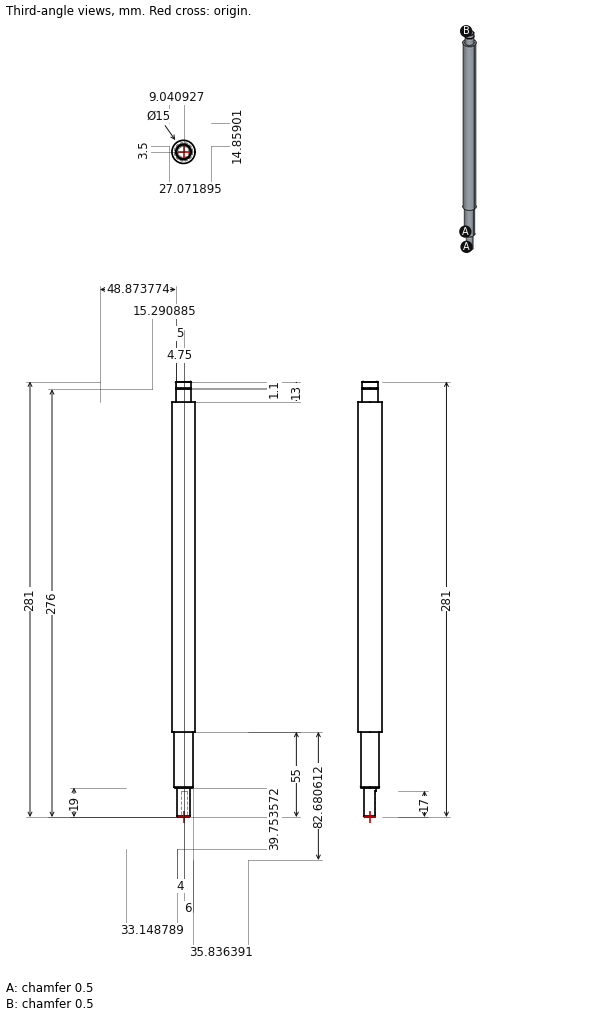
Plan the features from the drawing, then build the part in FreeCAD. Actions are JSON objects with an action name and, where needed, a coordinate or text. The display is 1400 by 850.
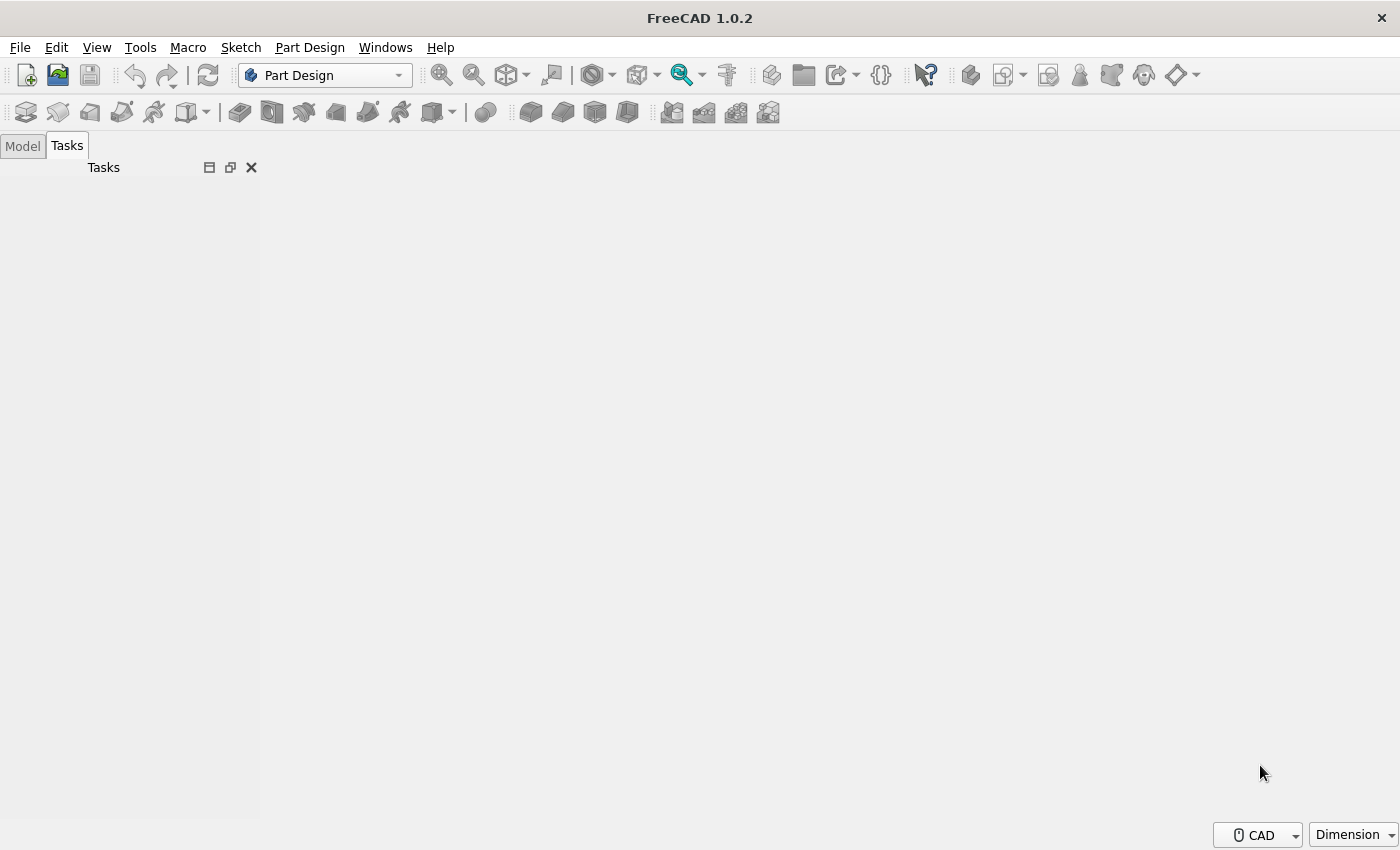
{"action": "left_click", "coordinate": [26, 76]}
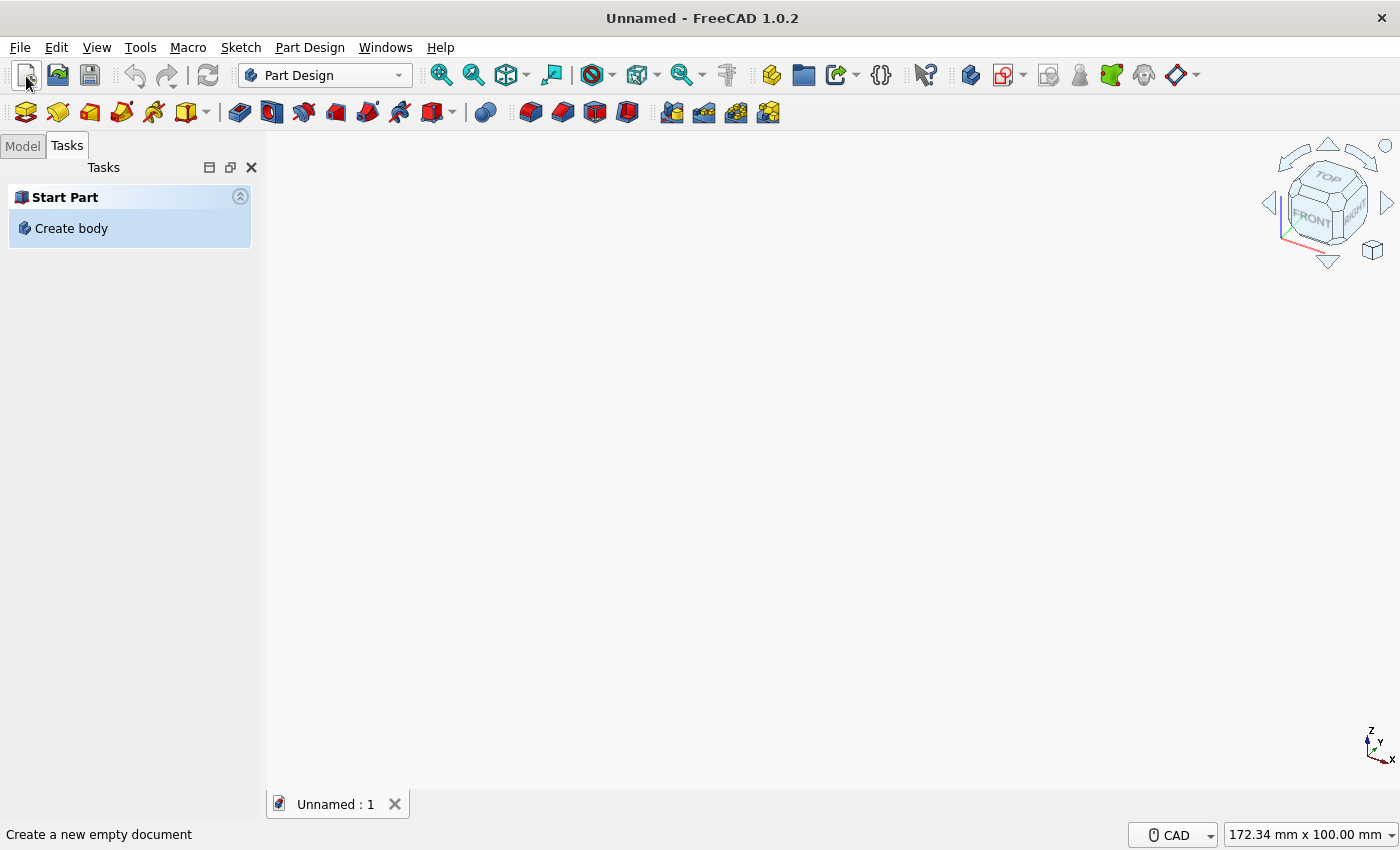
{"action": "left_click", "coordinate": [1004, 76]}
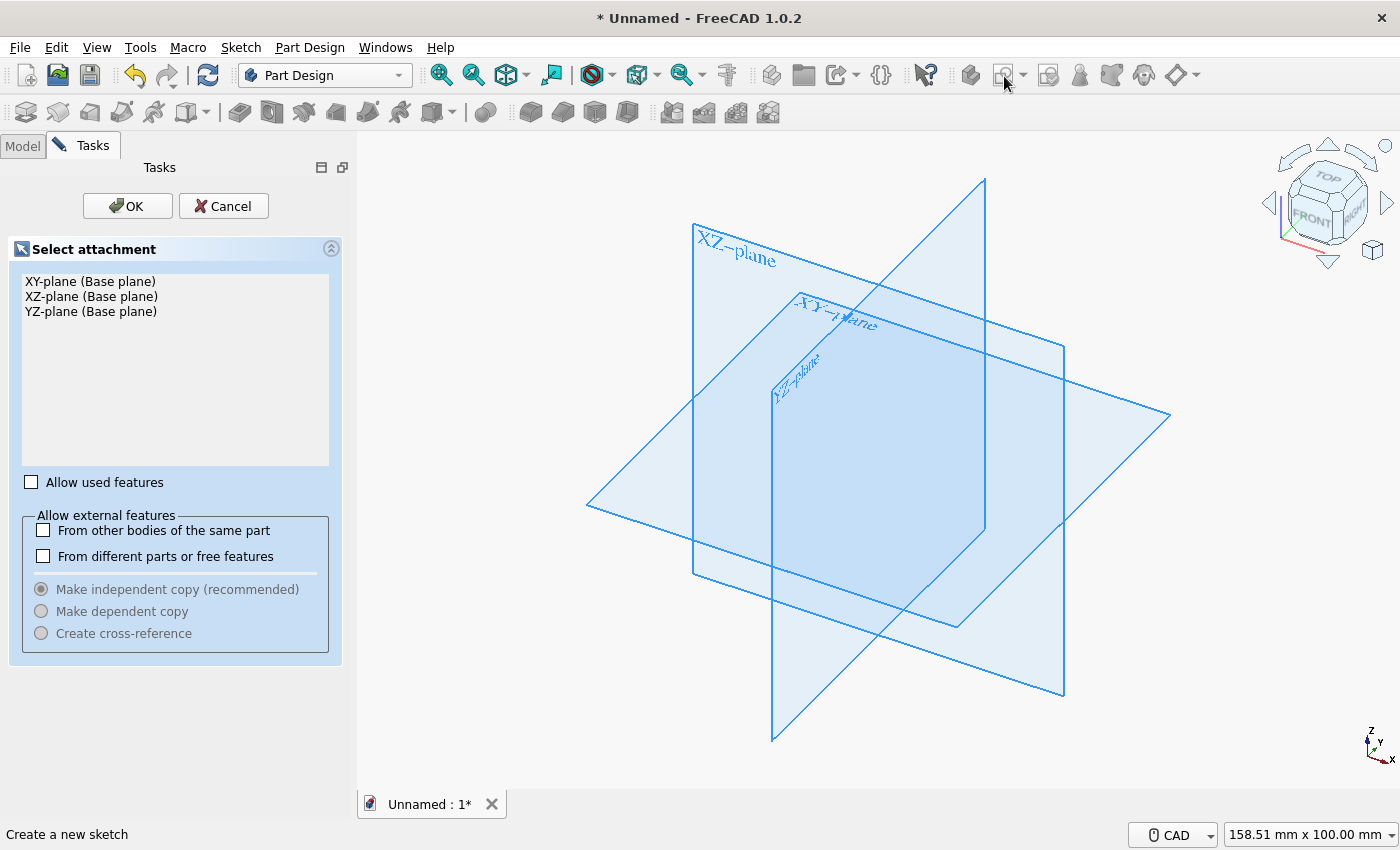
{"action": "left_click", "coordinate": [82, 282]}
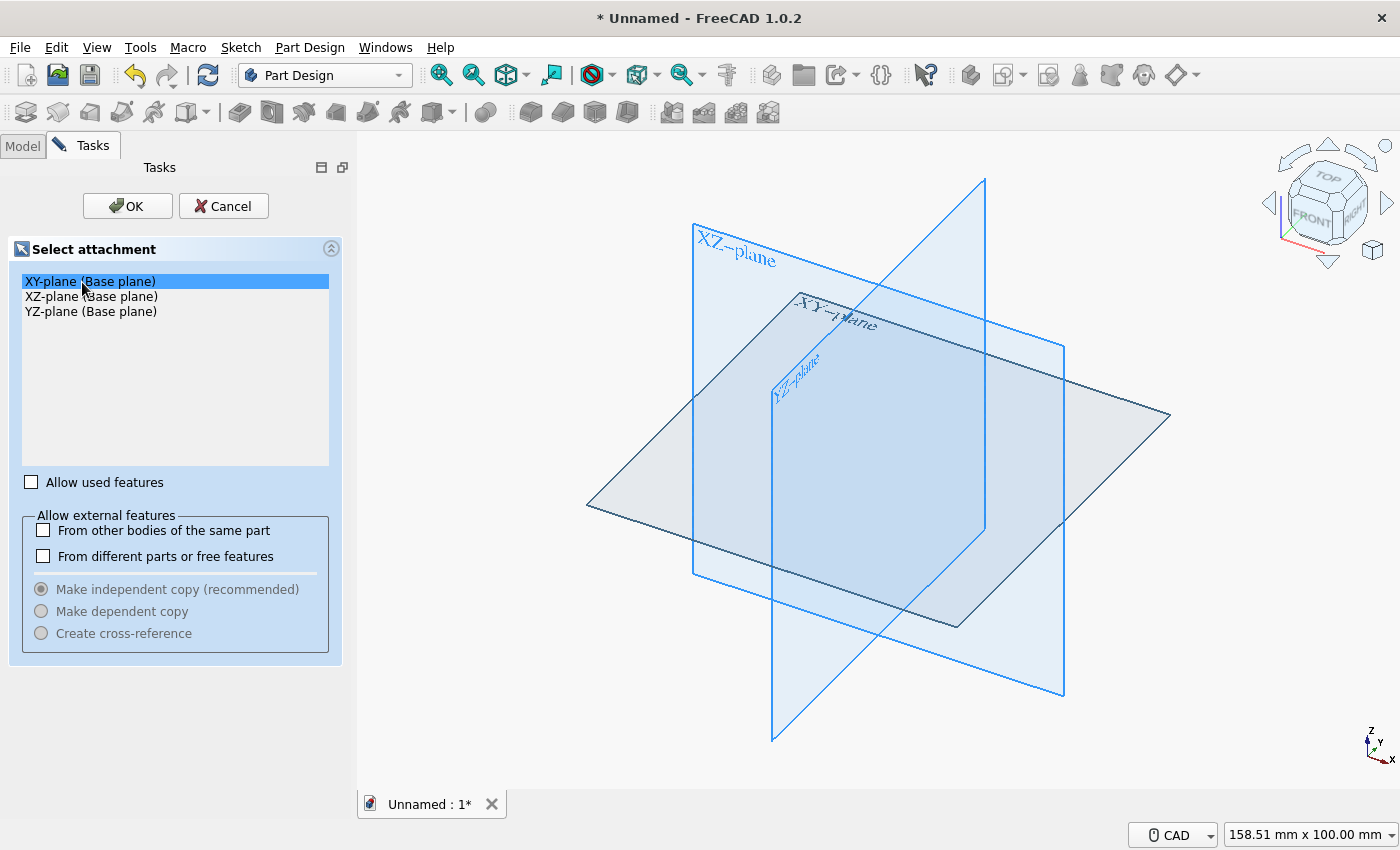
{"action": "left_click", "coordinate": [128, 206]}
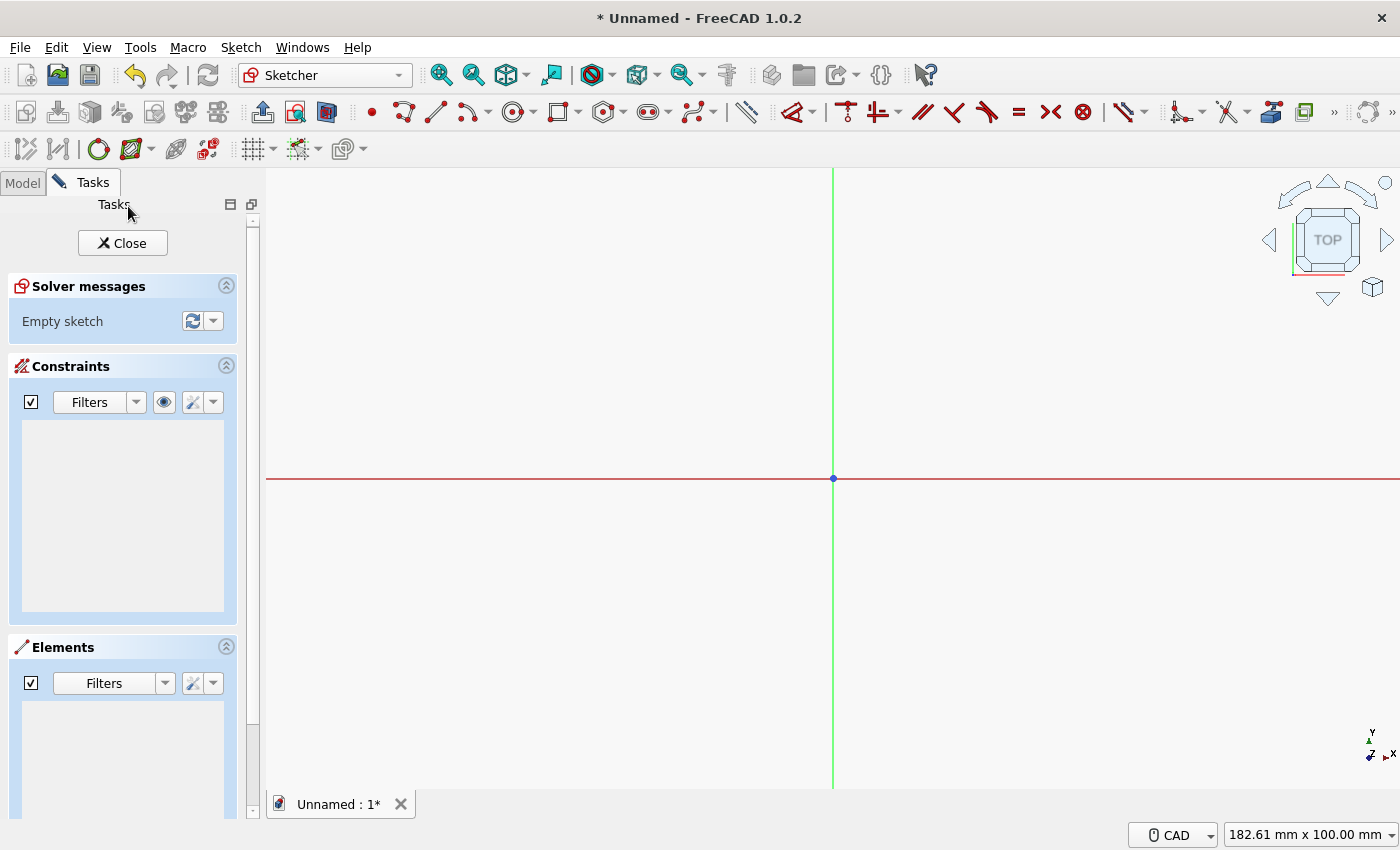
{"action": "scroll", "coordinate": [855, 479], "scroll_direction": "up", "scroll_amount": 7}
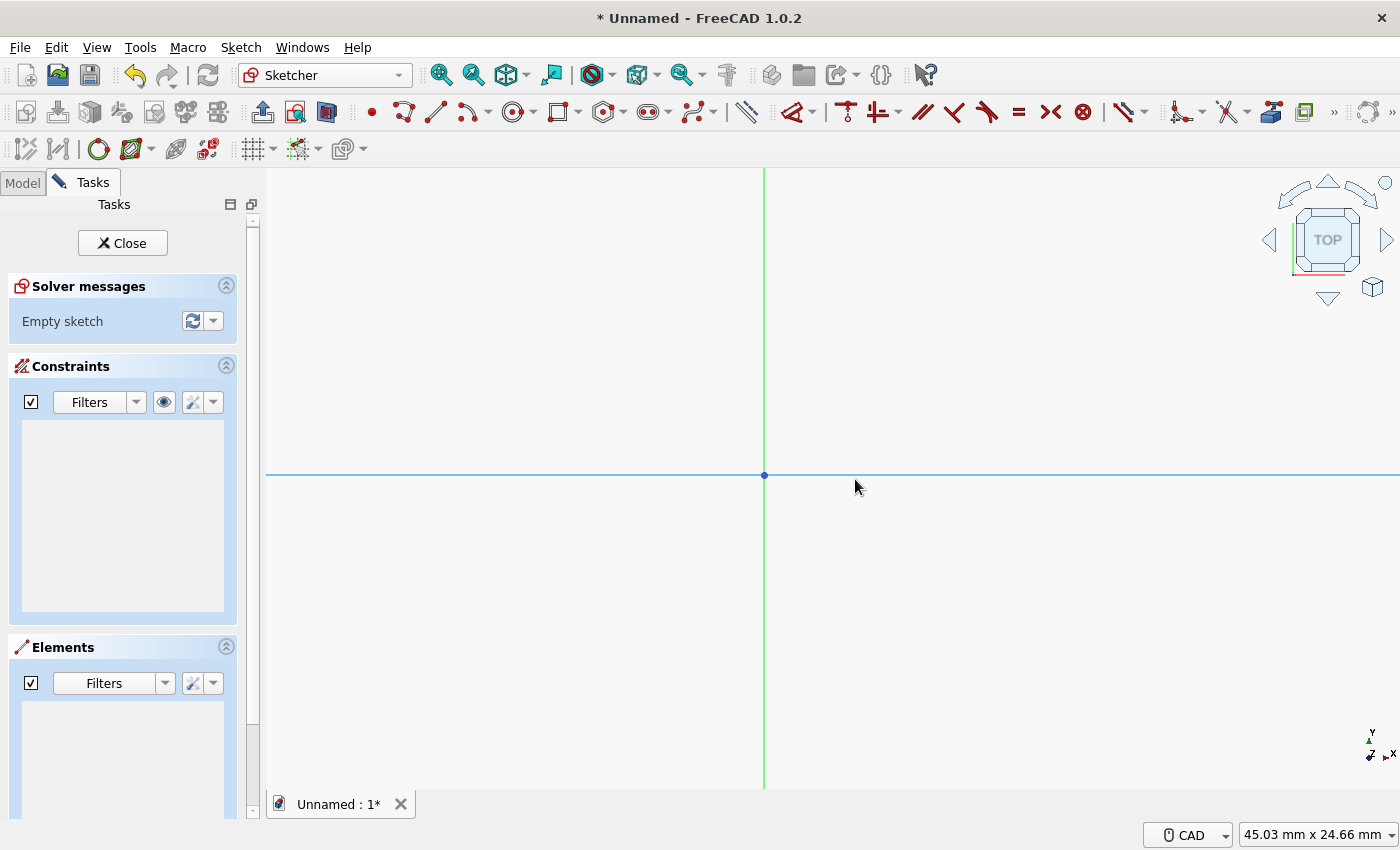
{"action": "left_click", "coordinate": [514, 112]}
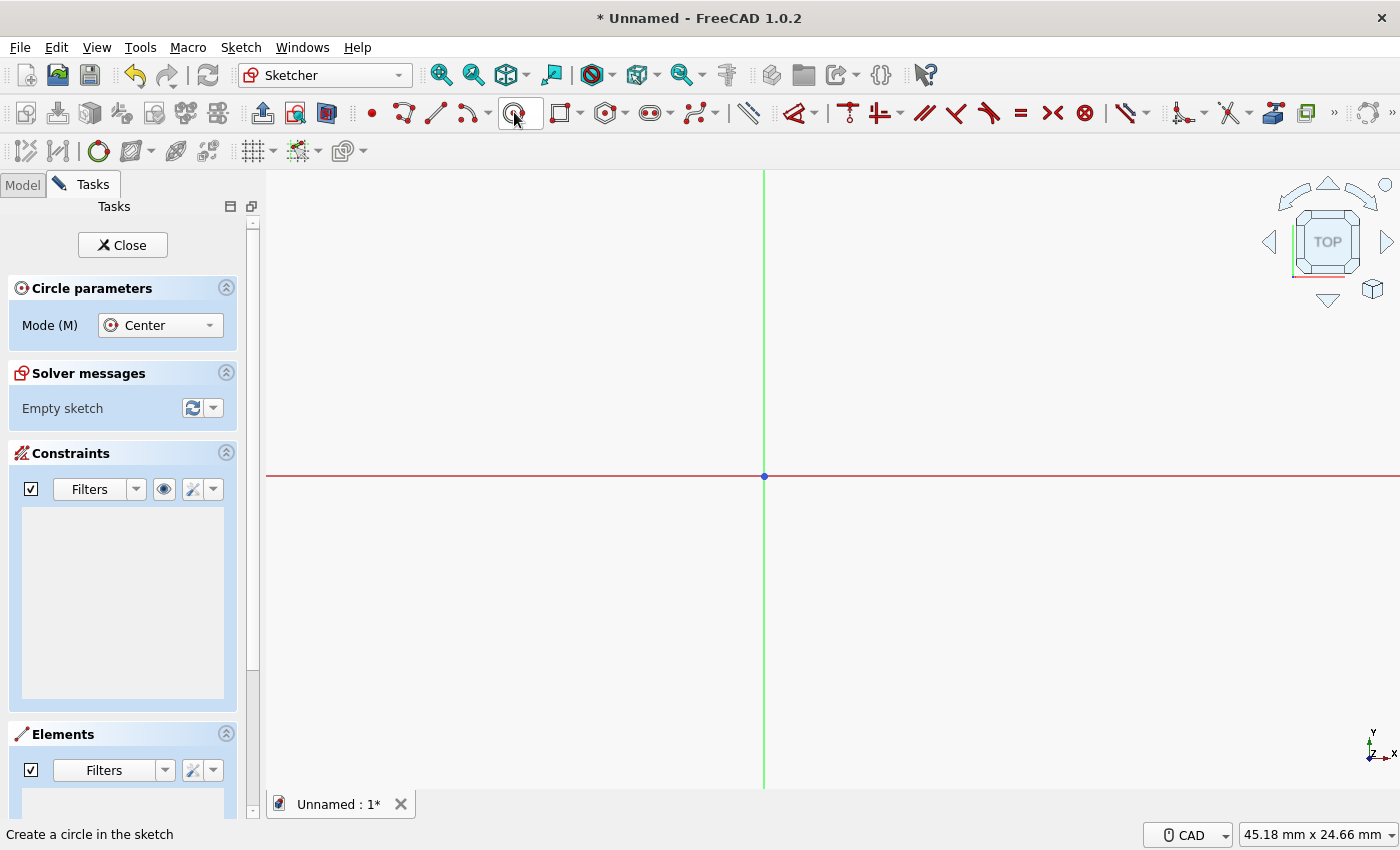
{"action": "left_click", "coordinate": [764, 476]}
{"action": "mouse_move", "coordinate": [898, 343]}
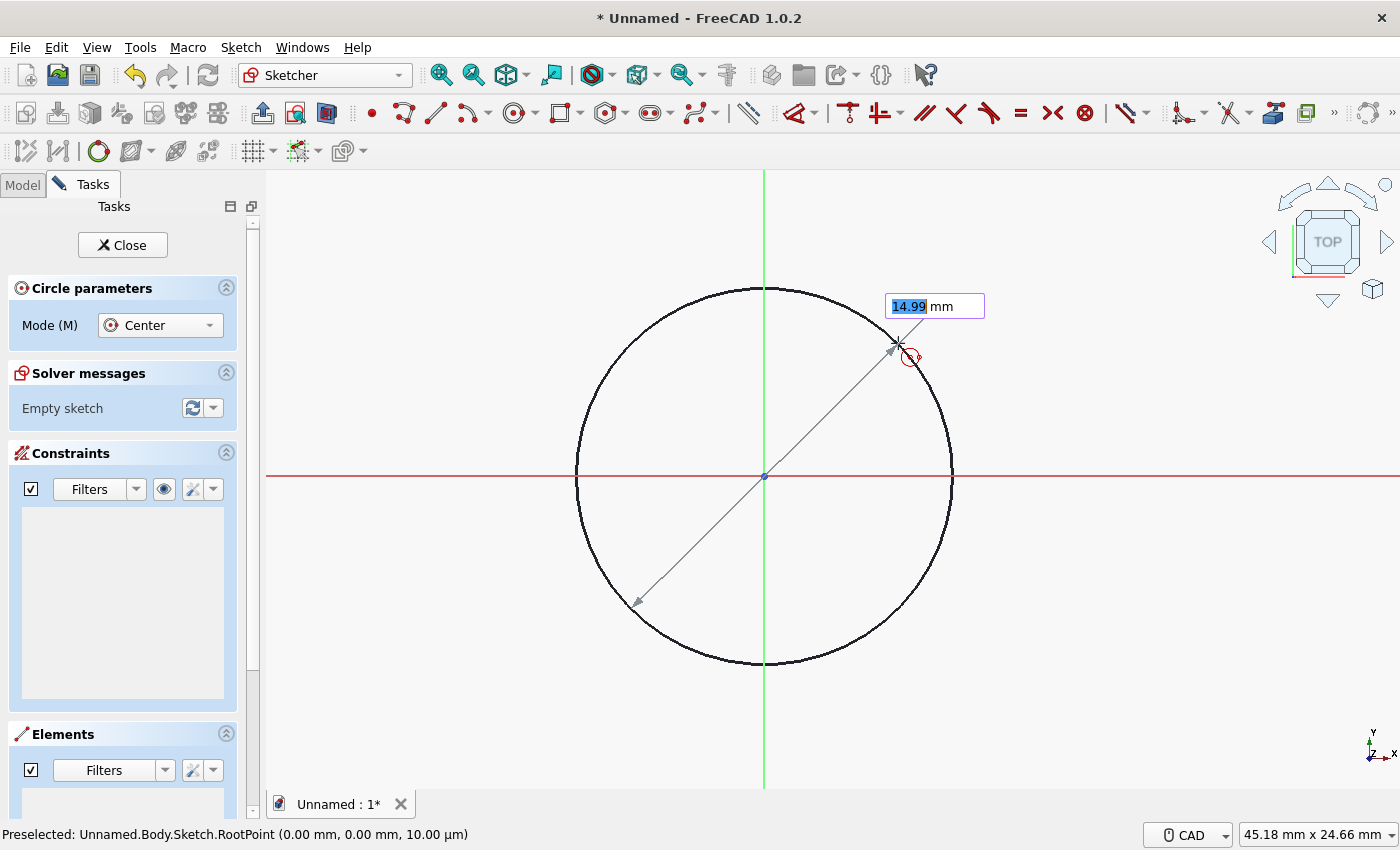
{"action": "type", "text": "15"}
{"action": "key", "text": "Return"}
{"action": "key", "text": "Escape"}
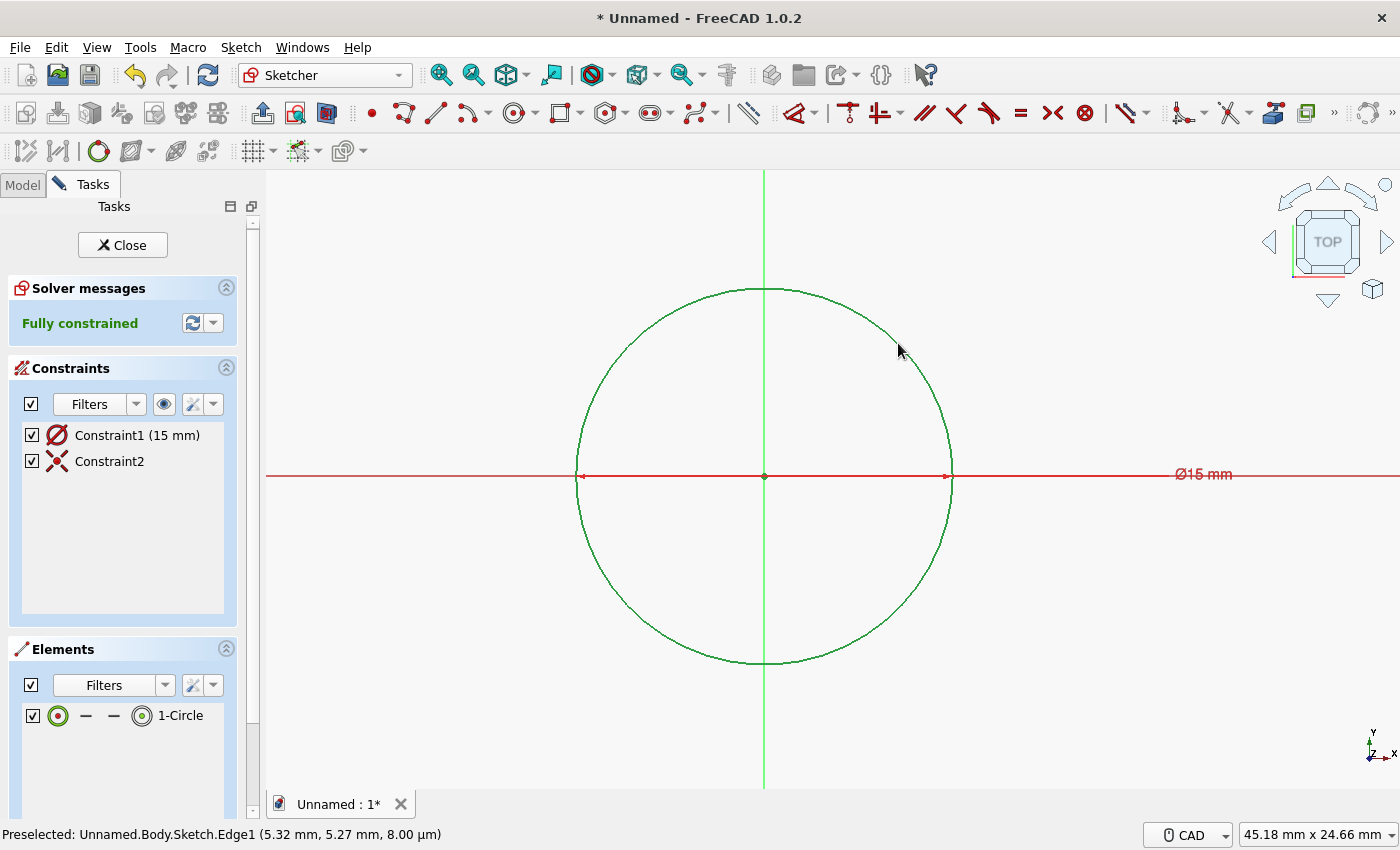
{"action": "left_click", "coordinate": [123, 245]}